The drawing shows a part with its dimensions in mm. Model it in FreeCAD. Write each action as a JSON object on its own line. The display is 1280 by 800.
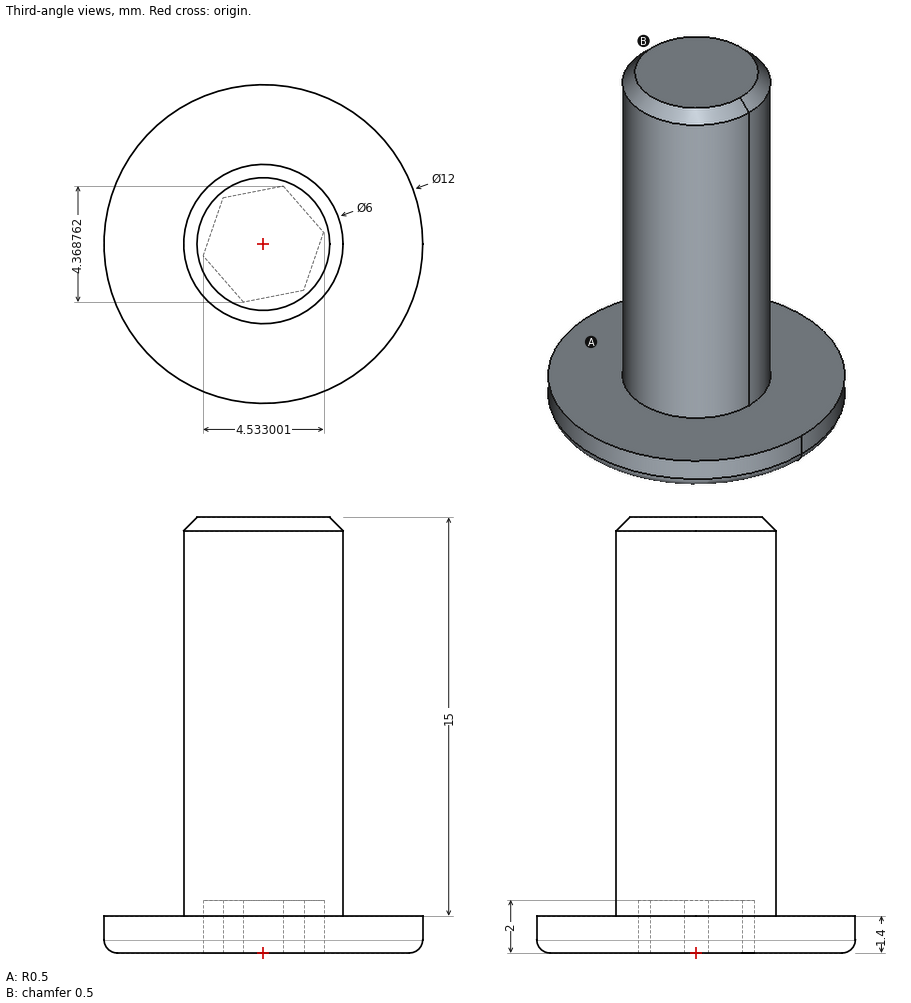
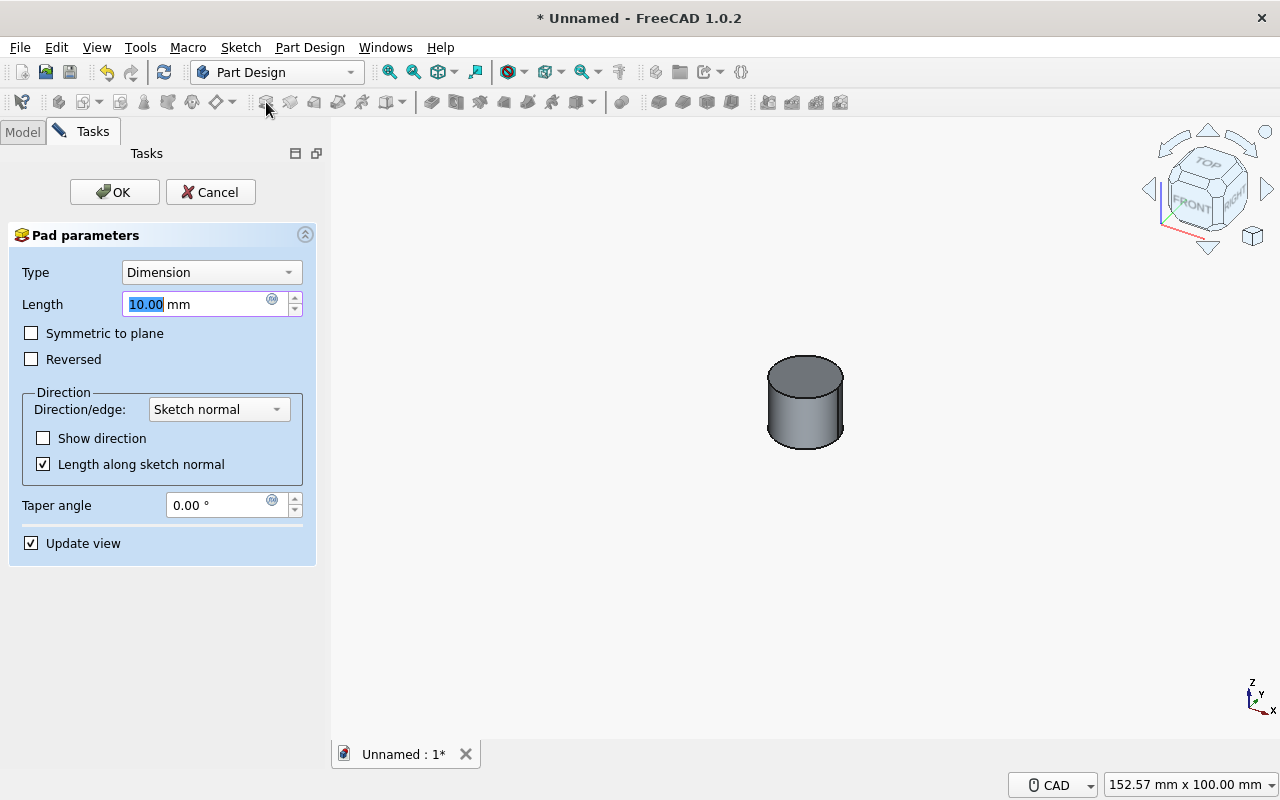
{"action": "type", "text": "1.4"}
{"action": "key", "text": "Tab"}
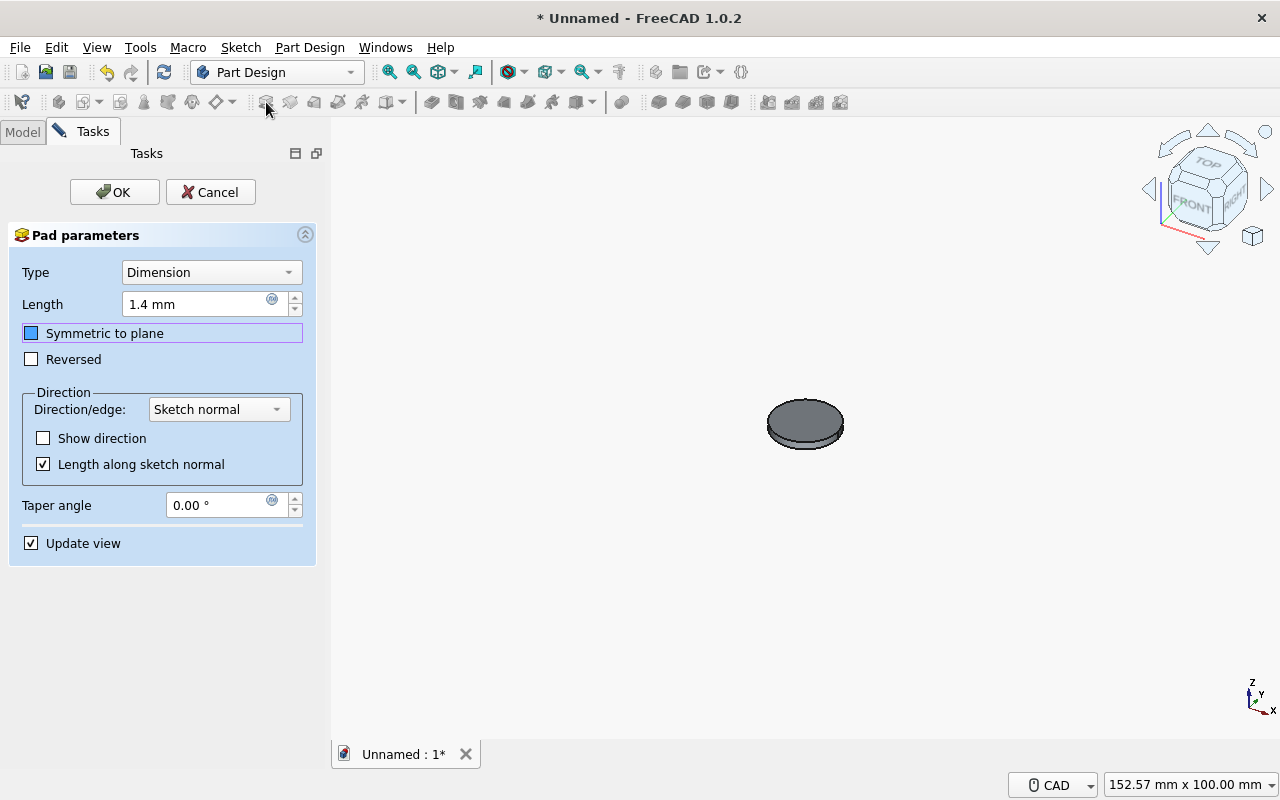
{"action": "left_click", "coordinate": [115, 192]}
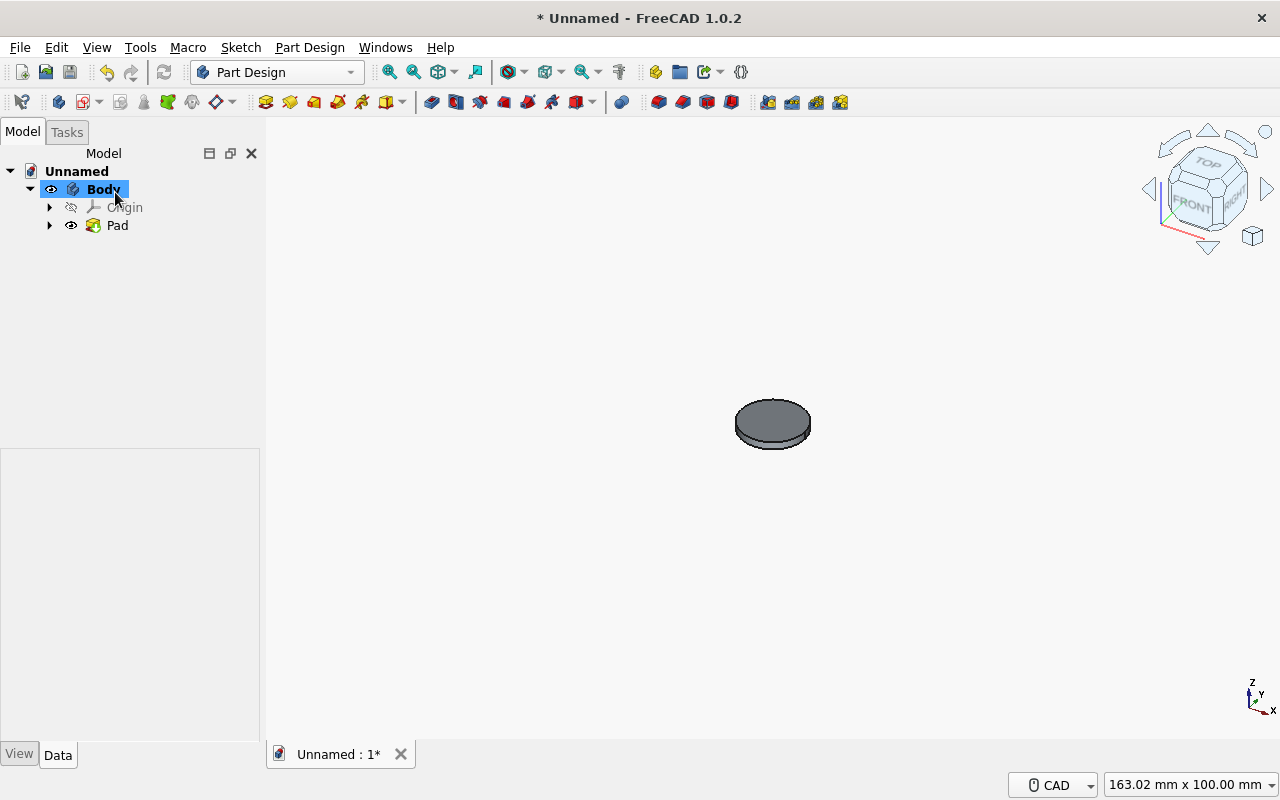
{"action": "left_click", "coordinate": [390, 72]}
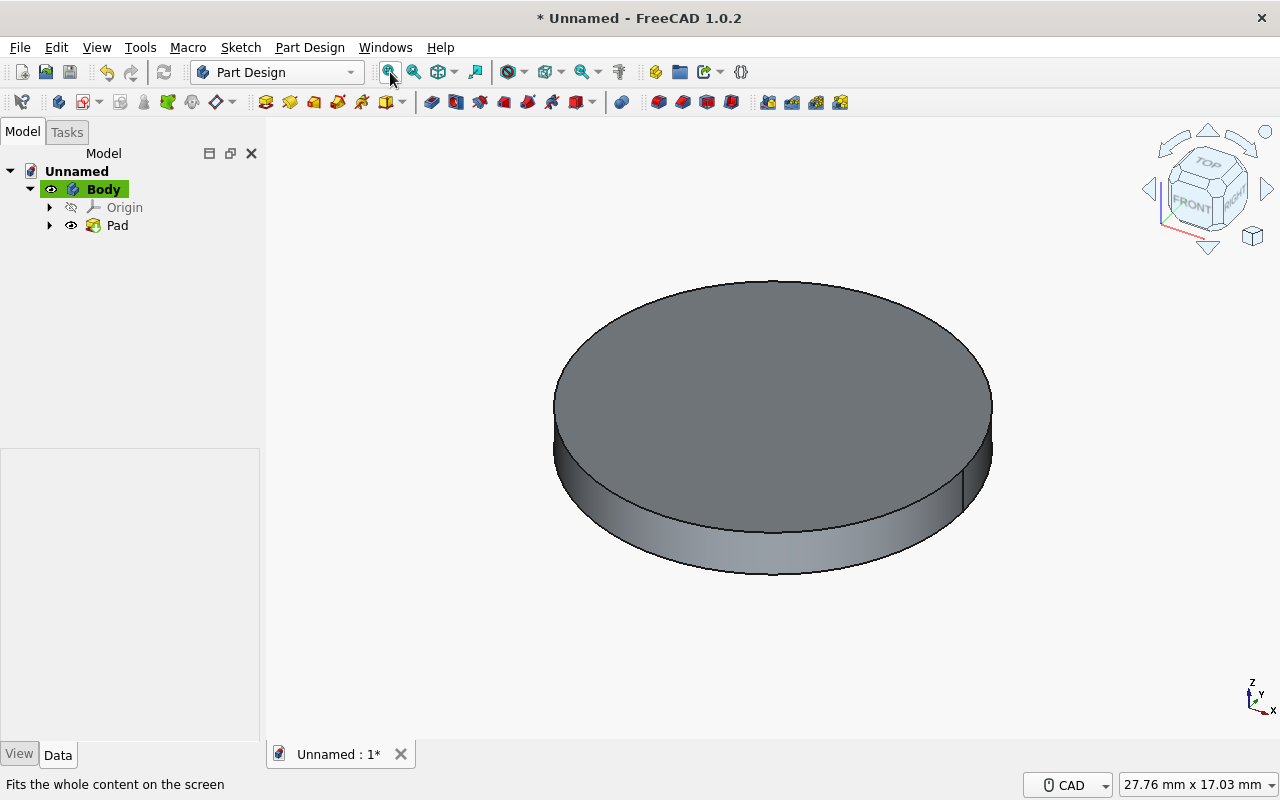
{"action": "left_click", "coordinate": [773, 406]}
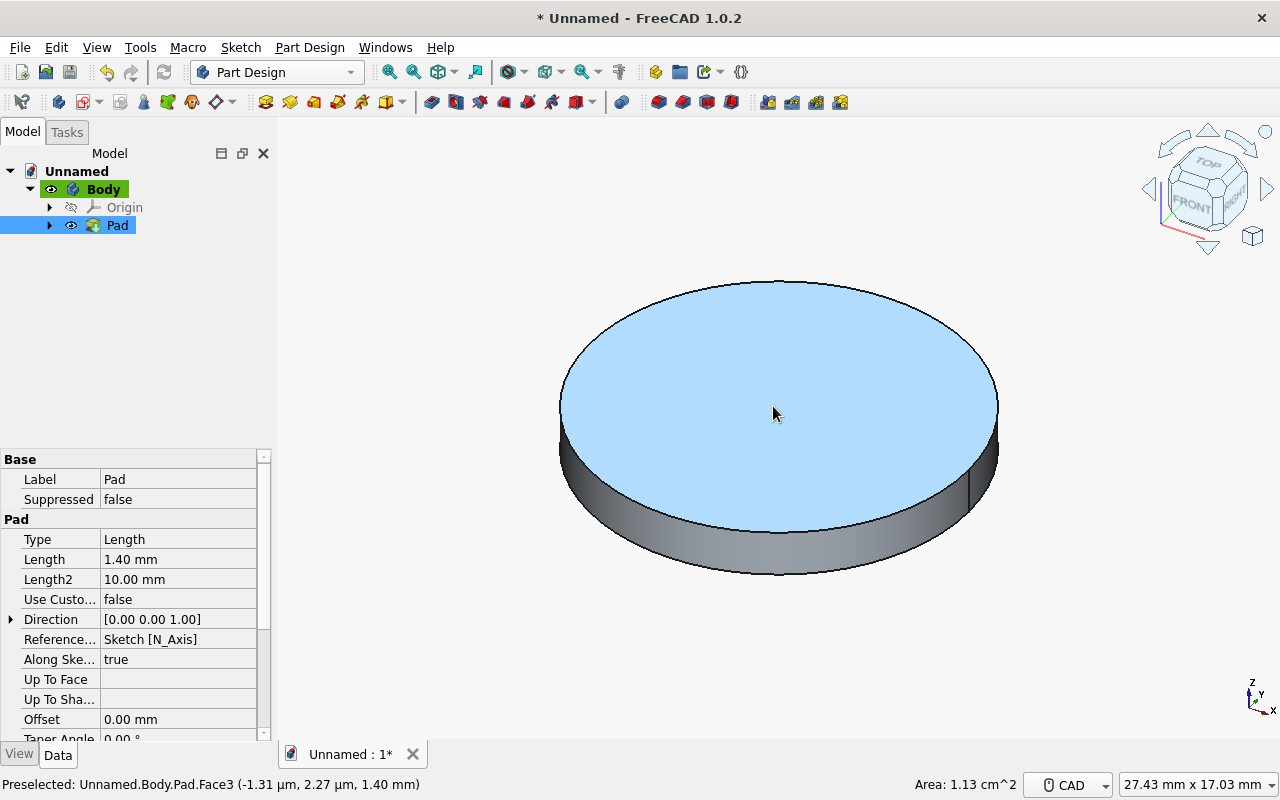
{"action": "left_click", "coordinate": [84, 102]}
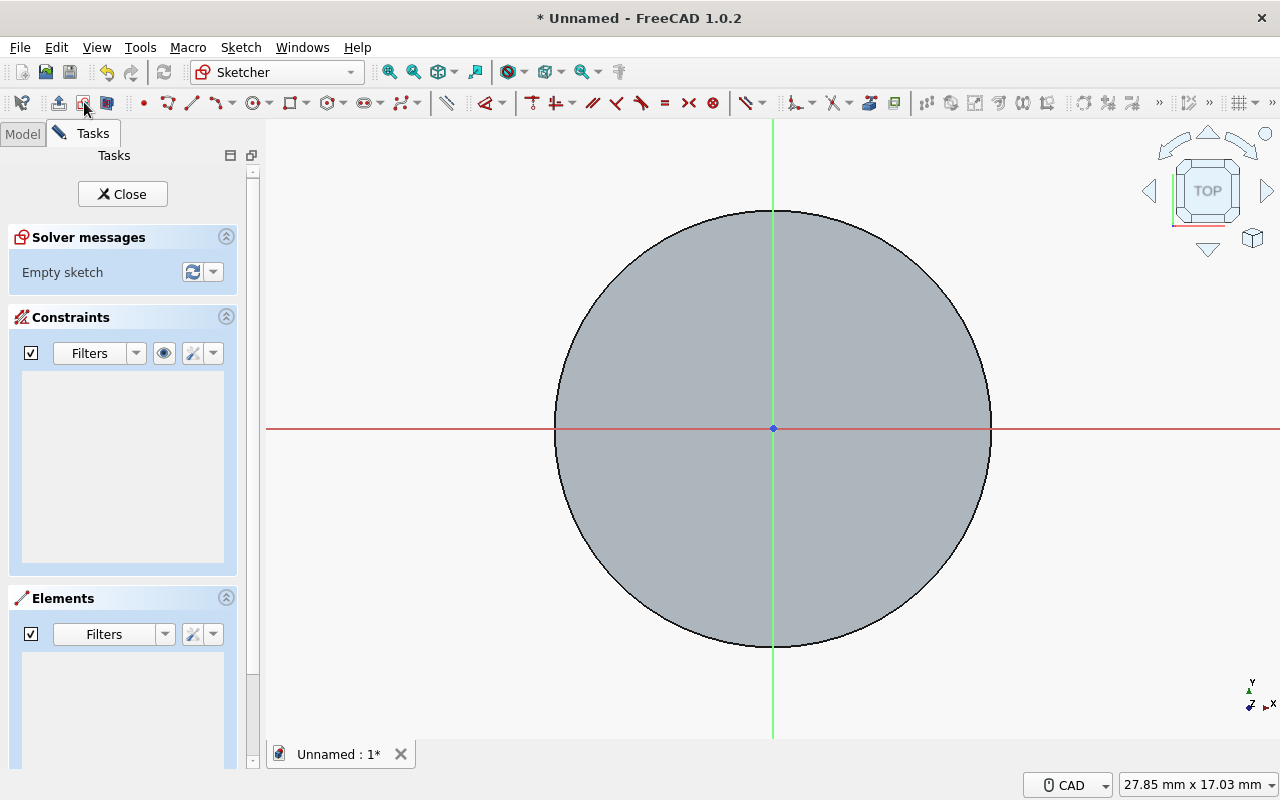
{"action": "scroll", "coordinate": [856, 429], "scroll_direction": "up", "scroll_amount": 3}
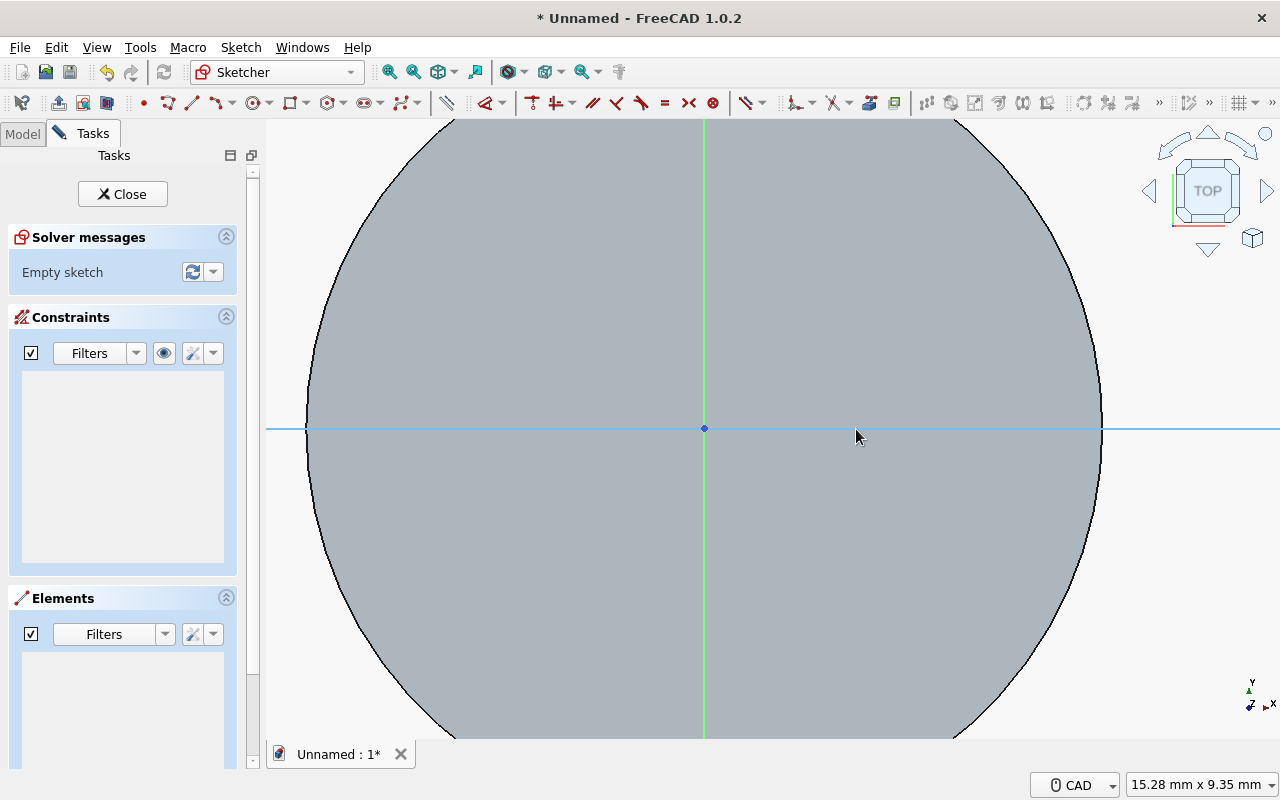
{"action": "left_click", "coordinate": [254, 104]}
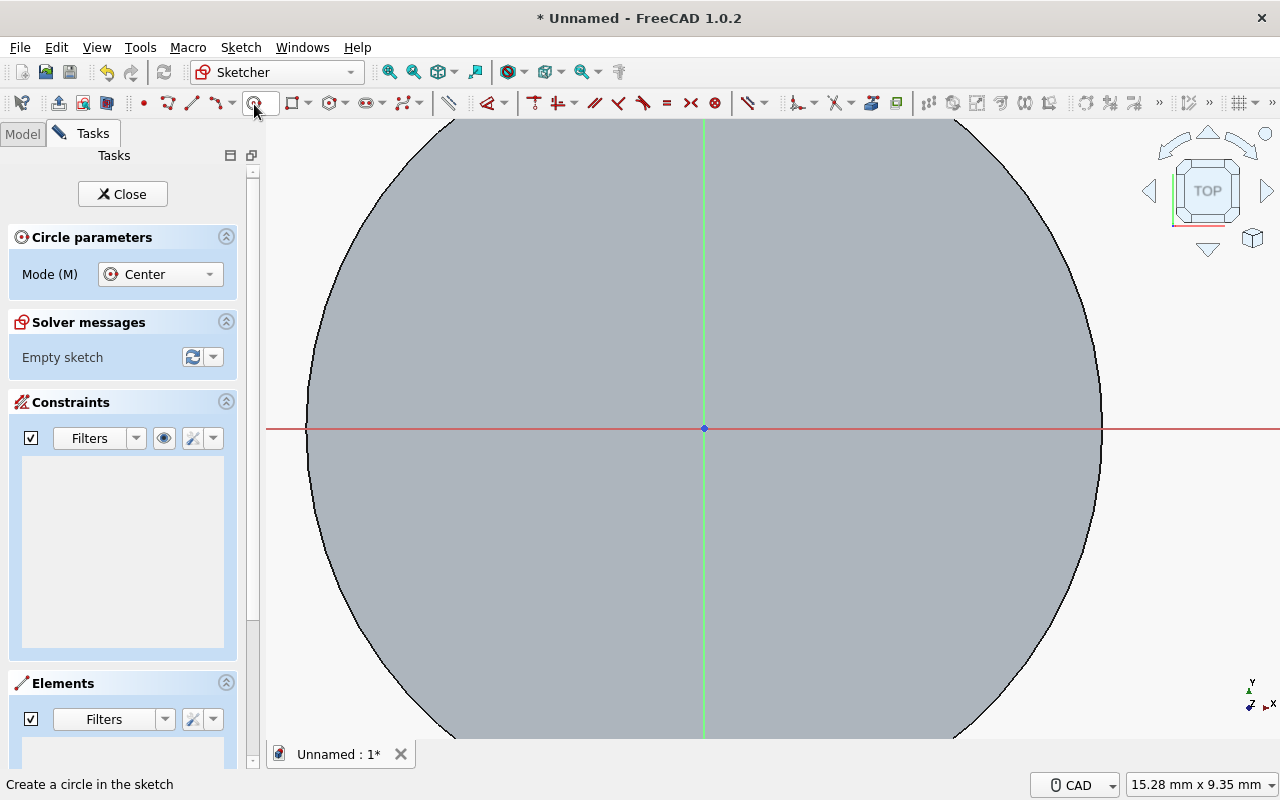
{"action": "left_click", "coordinate": [704, 429]}
{"action": "mouse_move", "coordinate": [845, 288]}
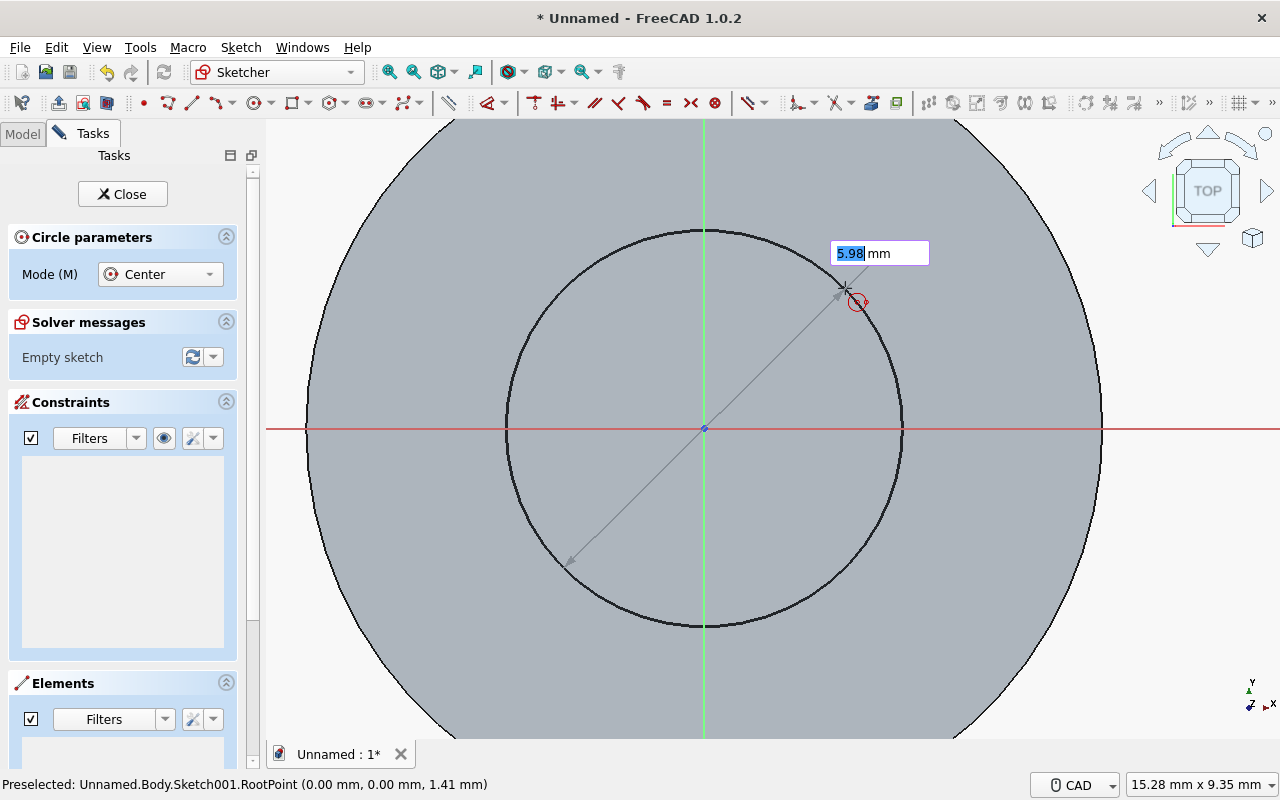
{"action": "type", "text": "6"}
{"action": "key", "text": "Return"}
{"action": "key", "text": "Escape"}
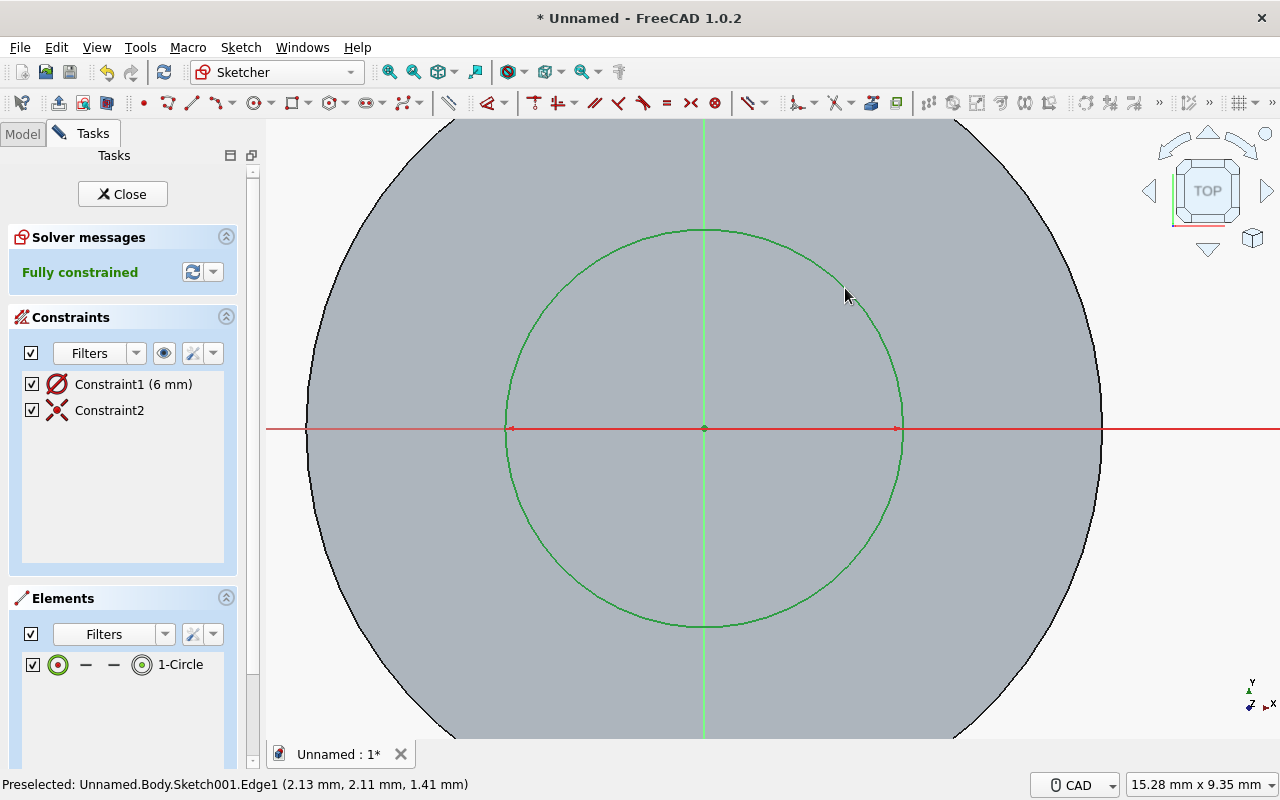
{"action": "left_click", "coordinate": [123, 194]}